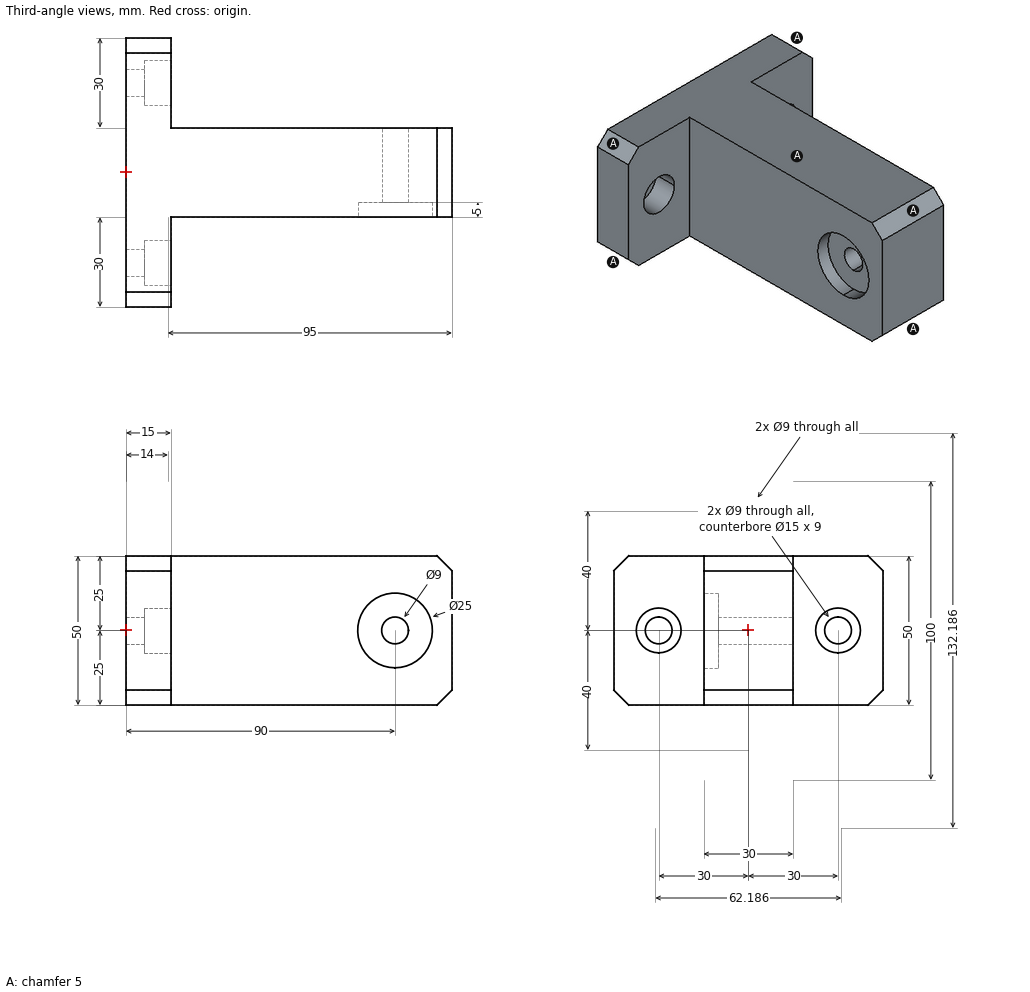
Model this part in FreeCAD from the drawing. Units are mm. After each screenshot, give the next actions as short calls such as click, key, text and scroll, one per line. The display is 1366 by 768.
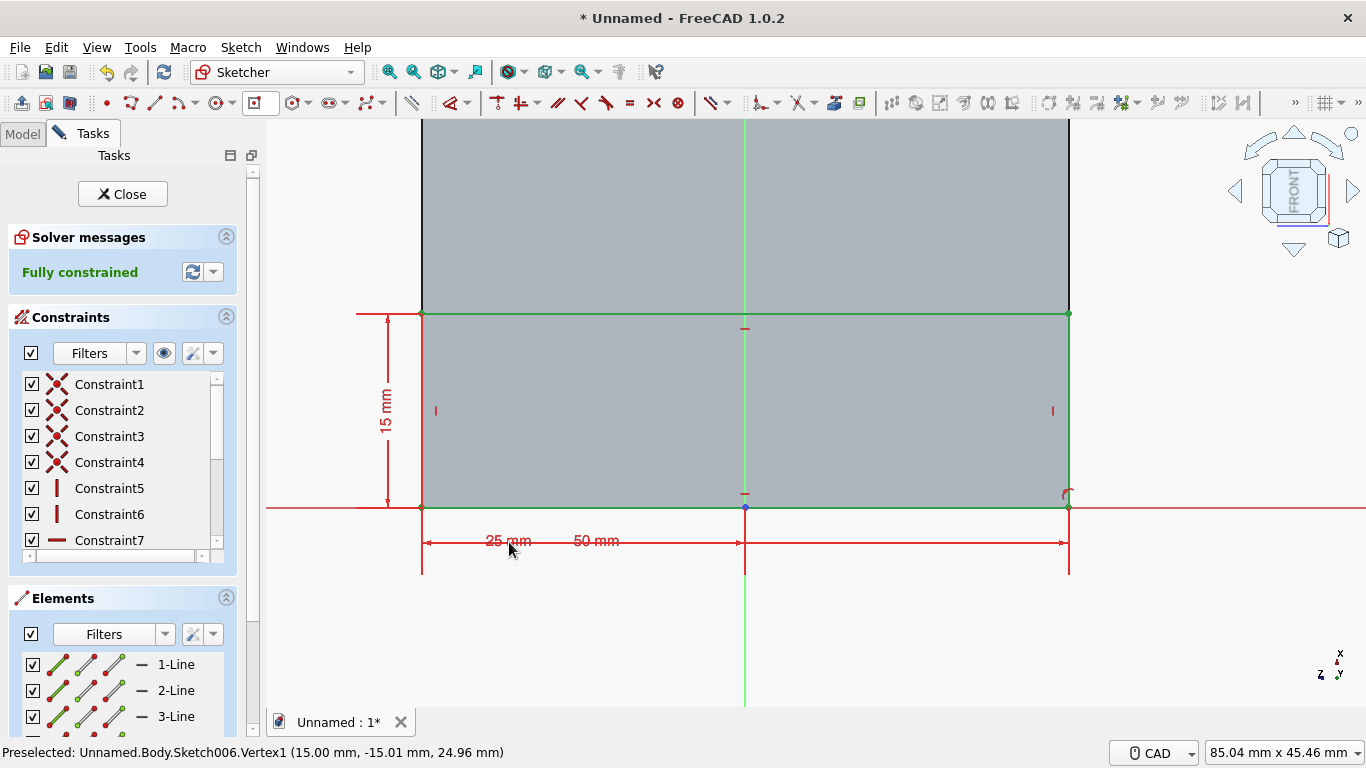
click(123, 194)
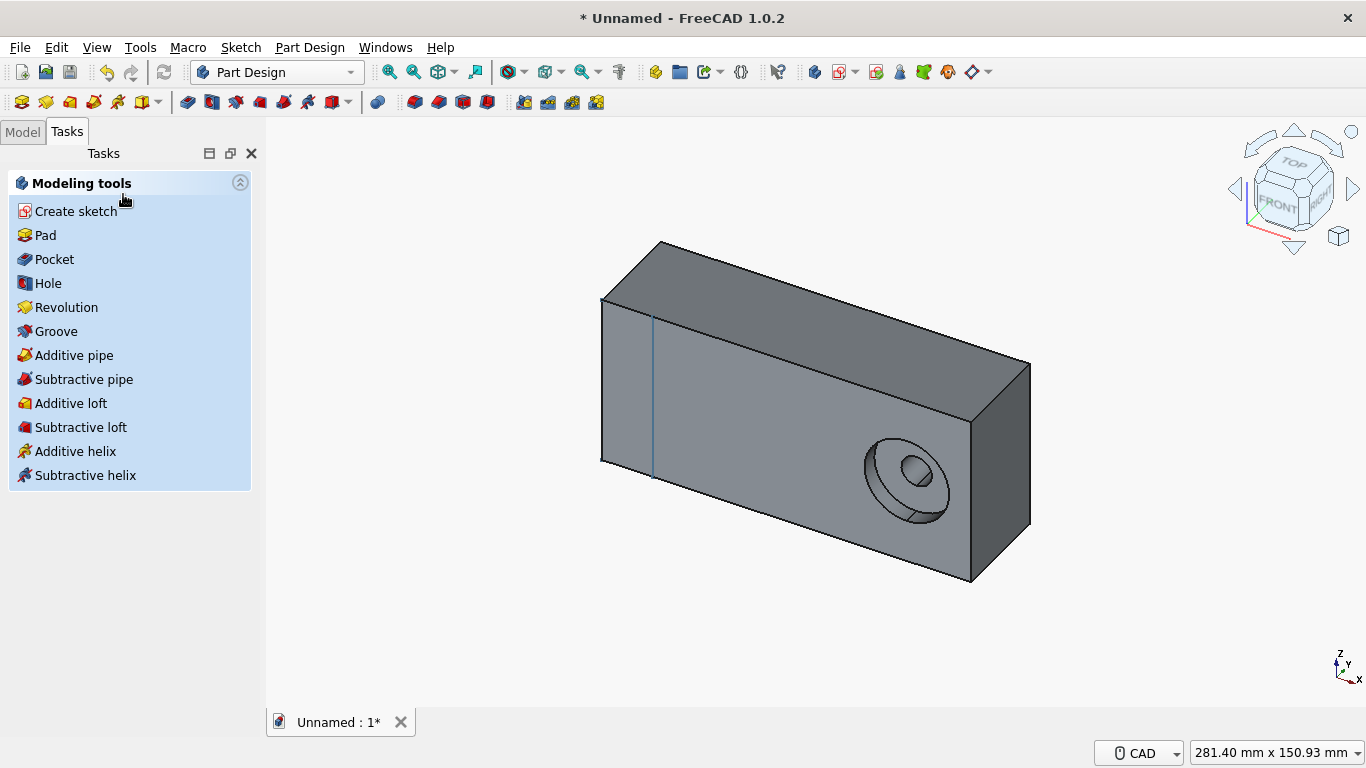
click(22, 102)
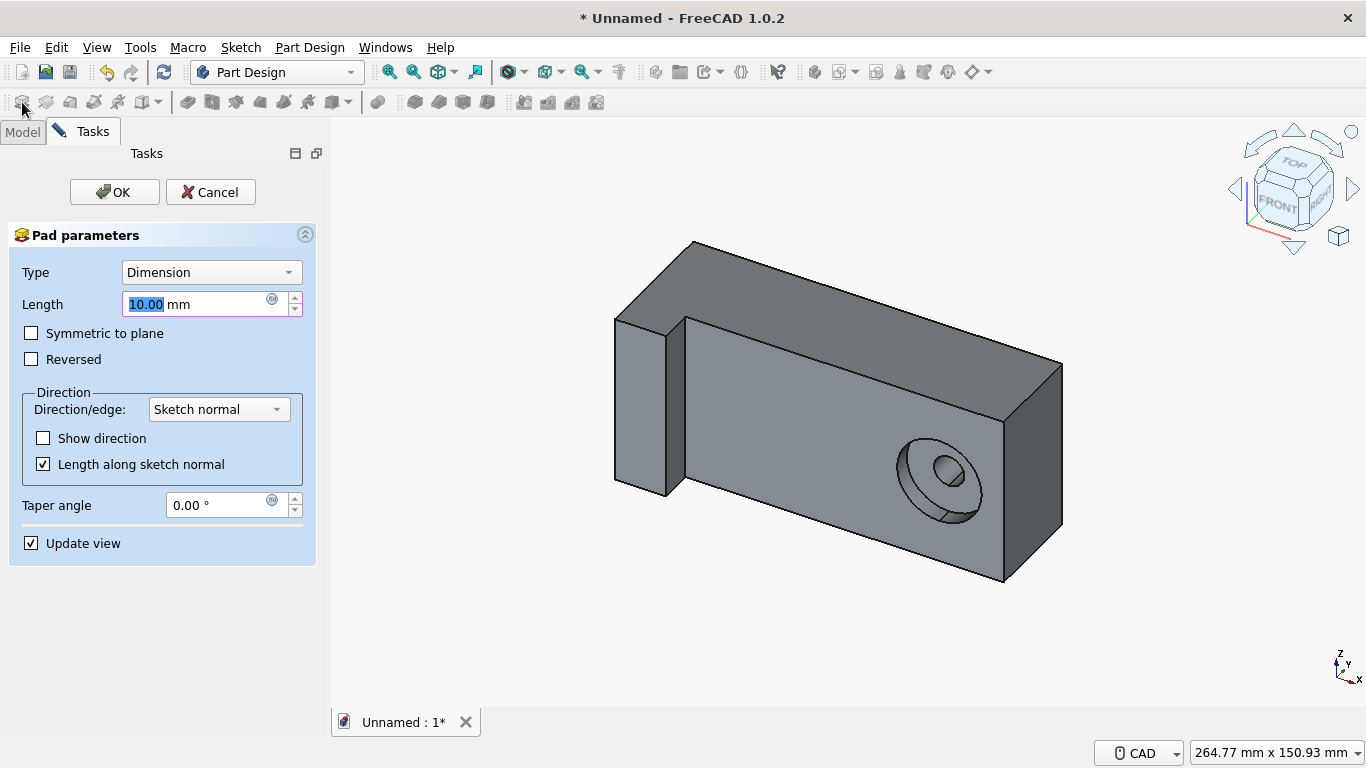
text(30)
key(Tab)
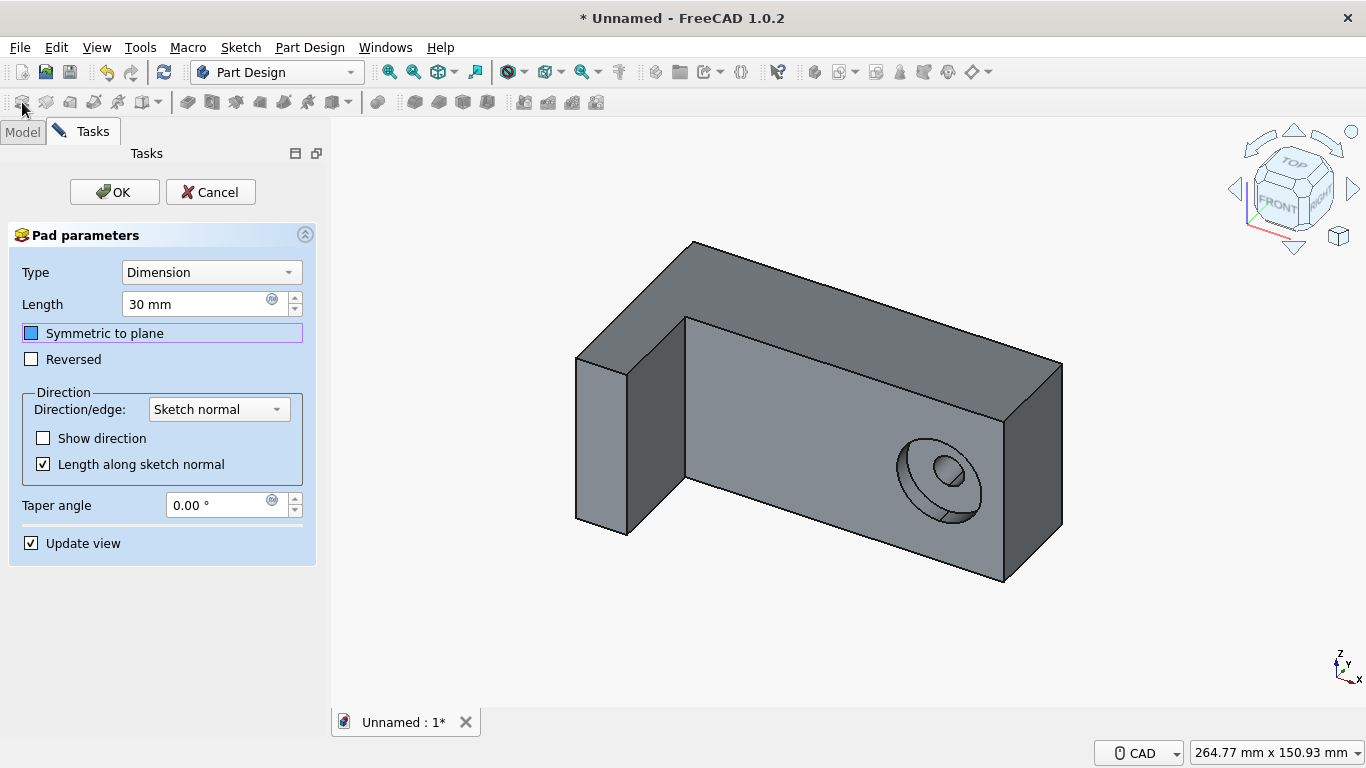
click(115, 192)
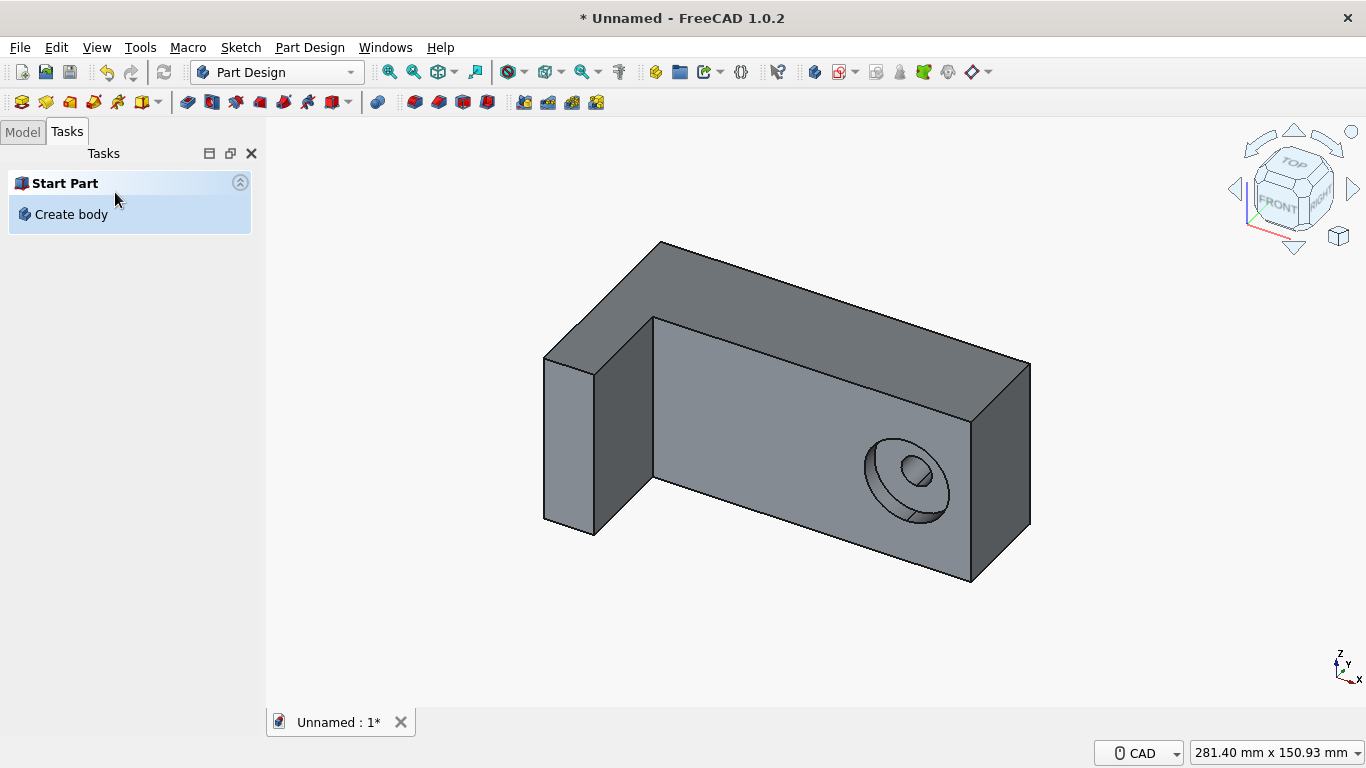
key(4)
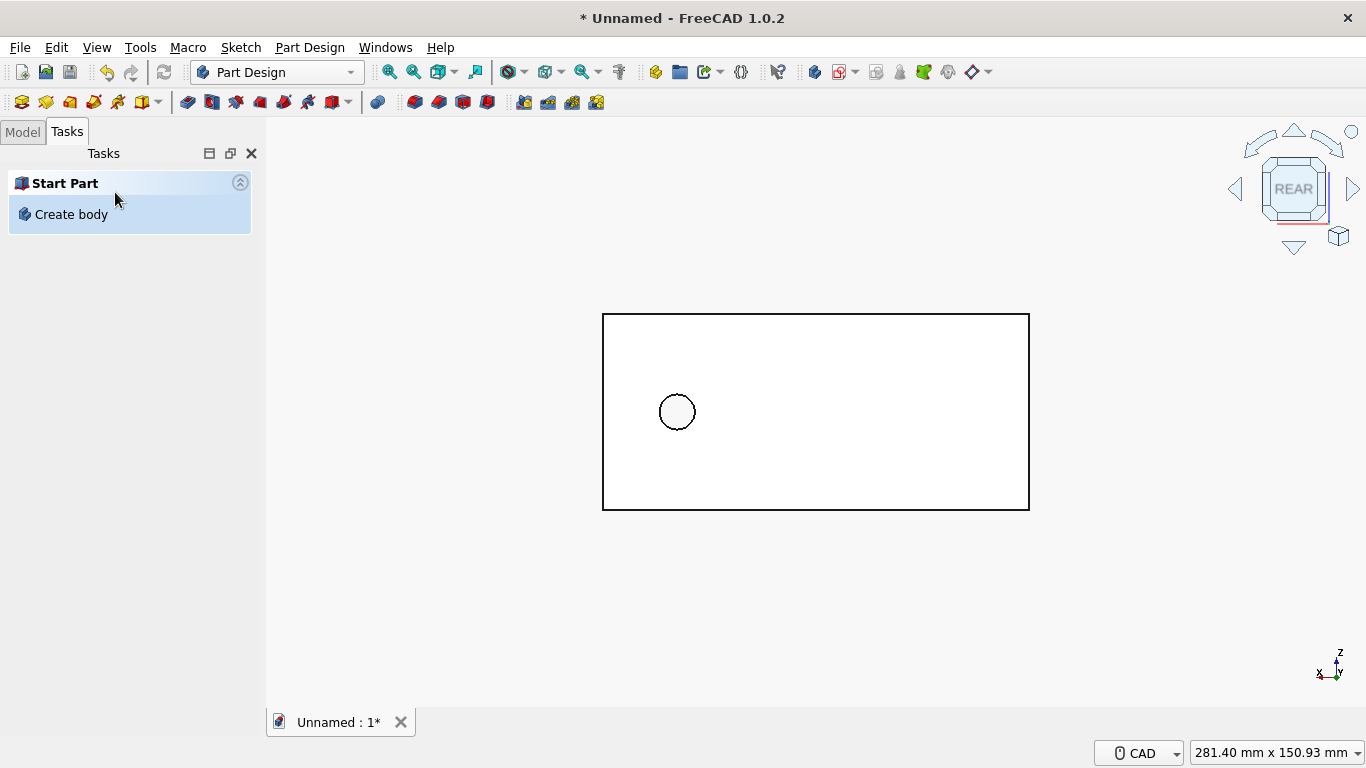
click(390, 72)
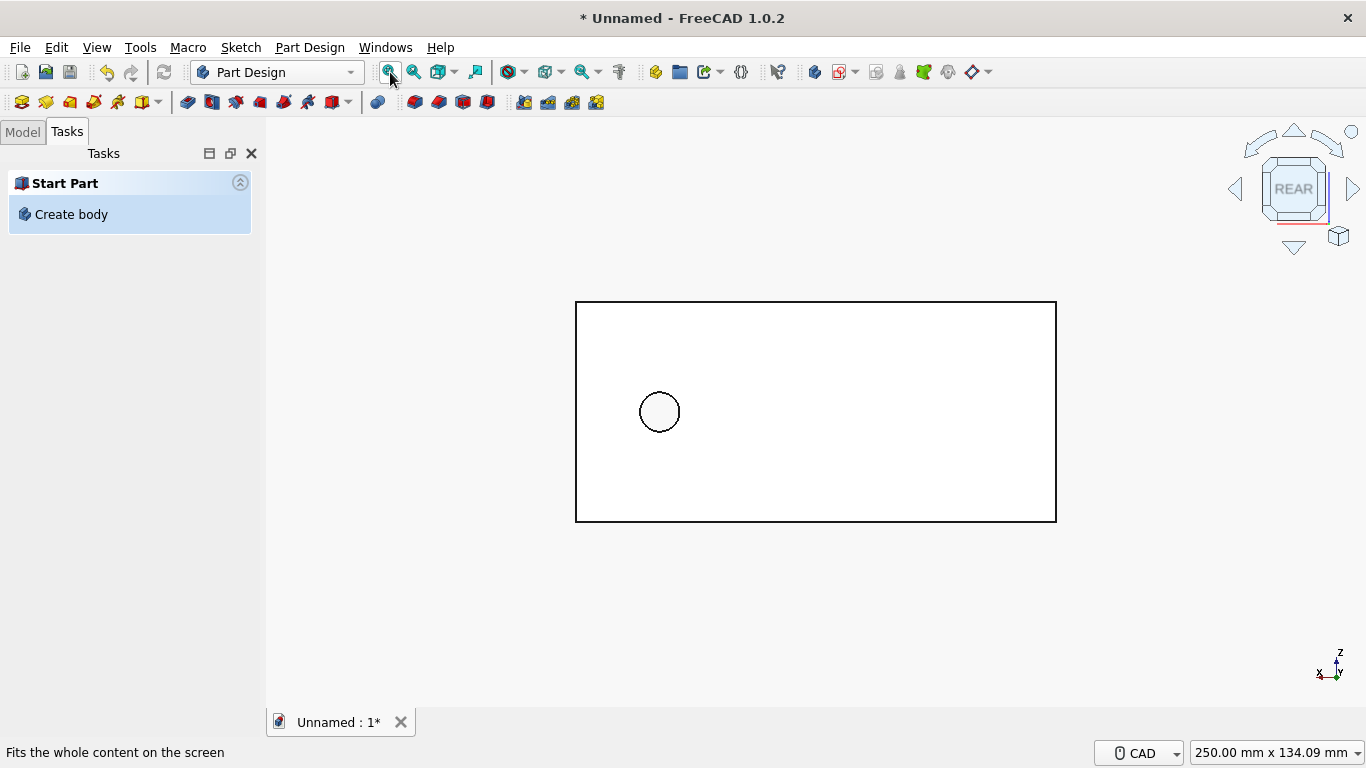
click(816, 411)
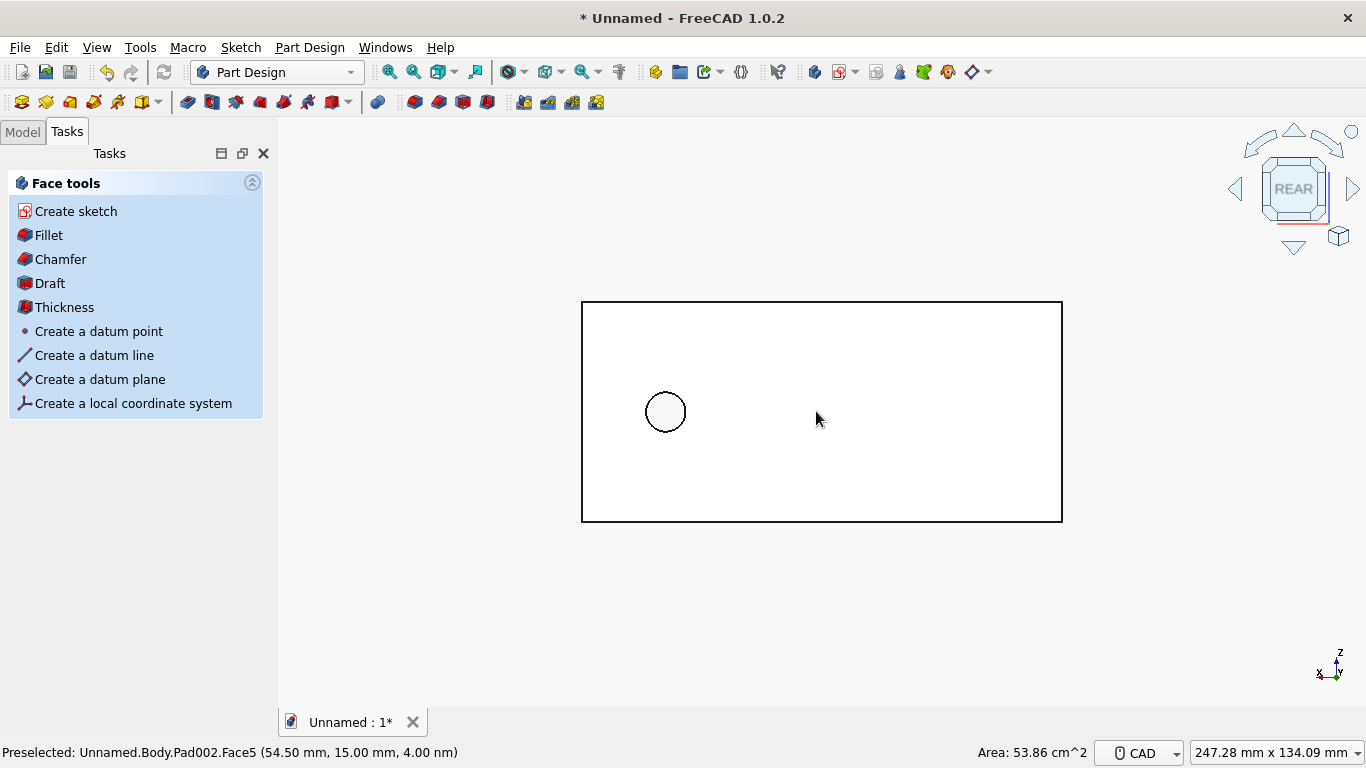
click(840, 72)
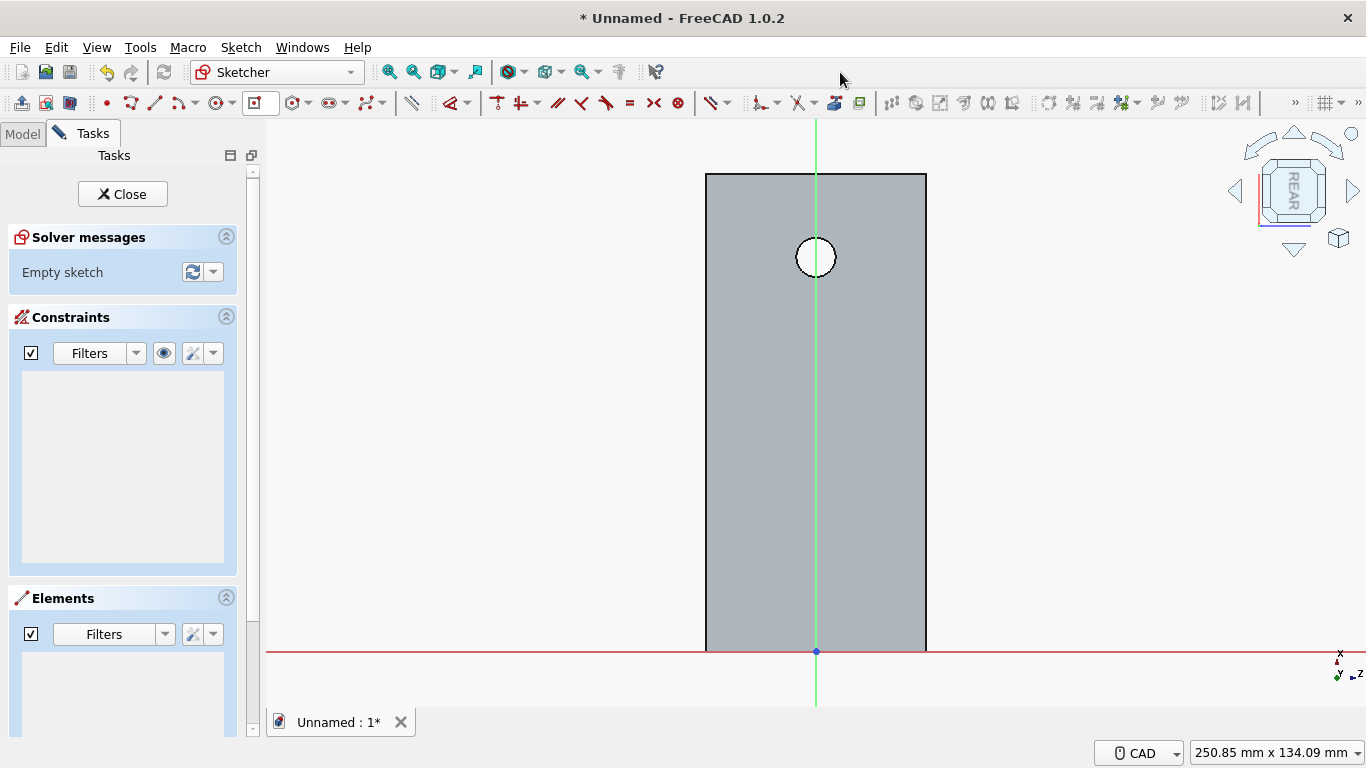
scroll(856, 679, up, 5)